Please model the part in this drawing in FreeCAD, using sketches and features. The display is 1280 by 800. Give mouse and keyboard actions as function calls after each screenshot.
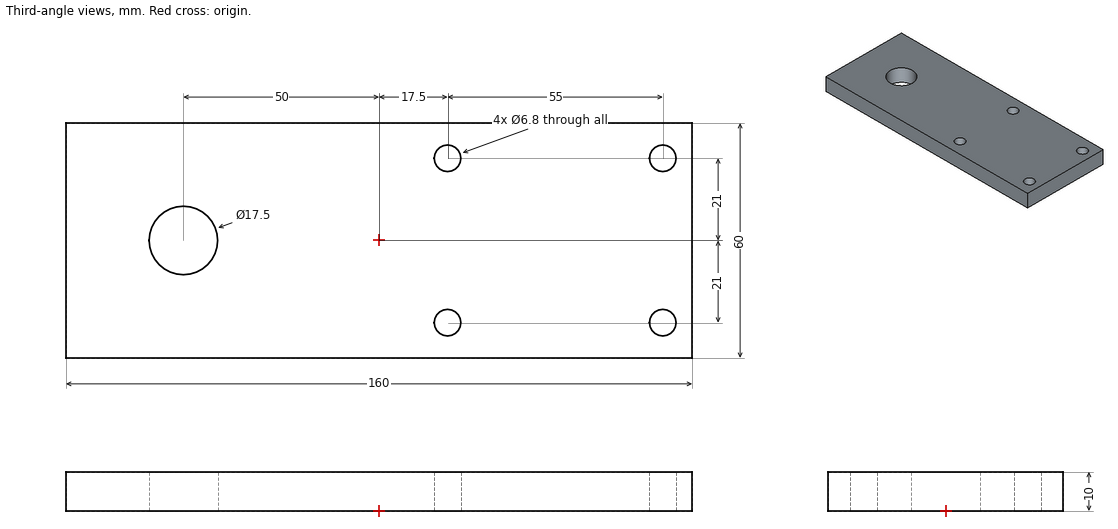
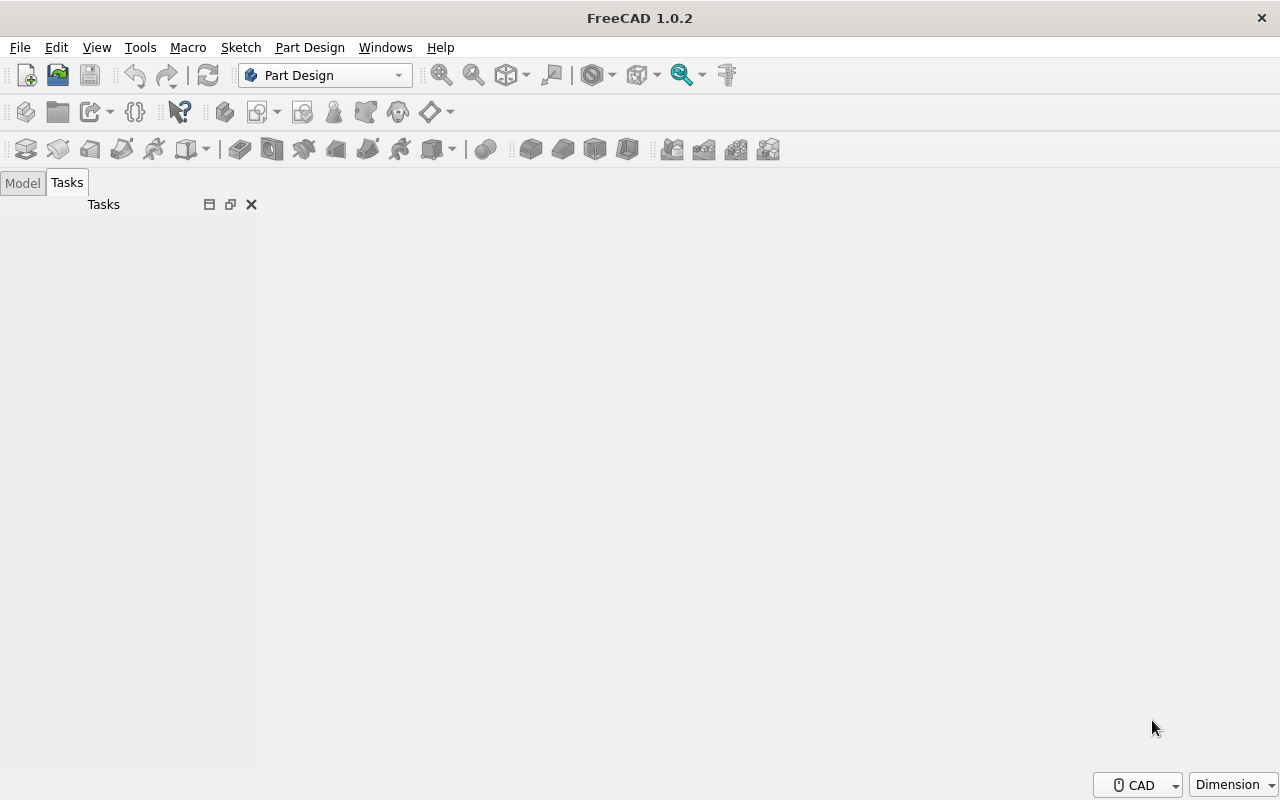
click(26, 76)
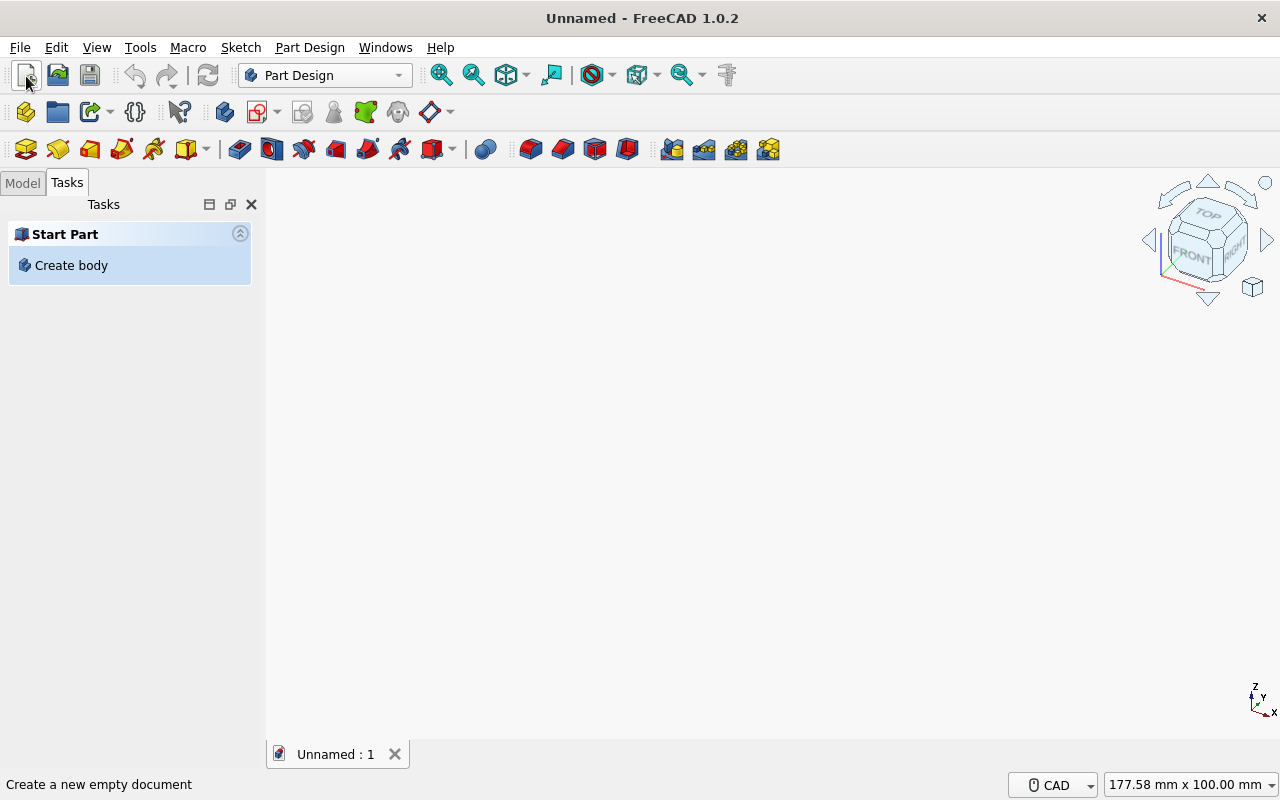
click(258, 112)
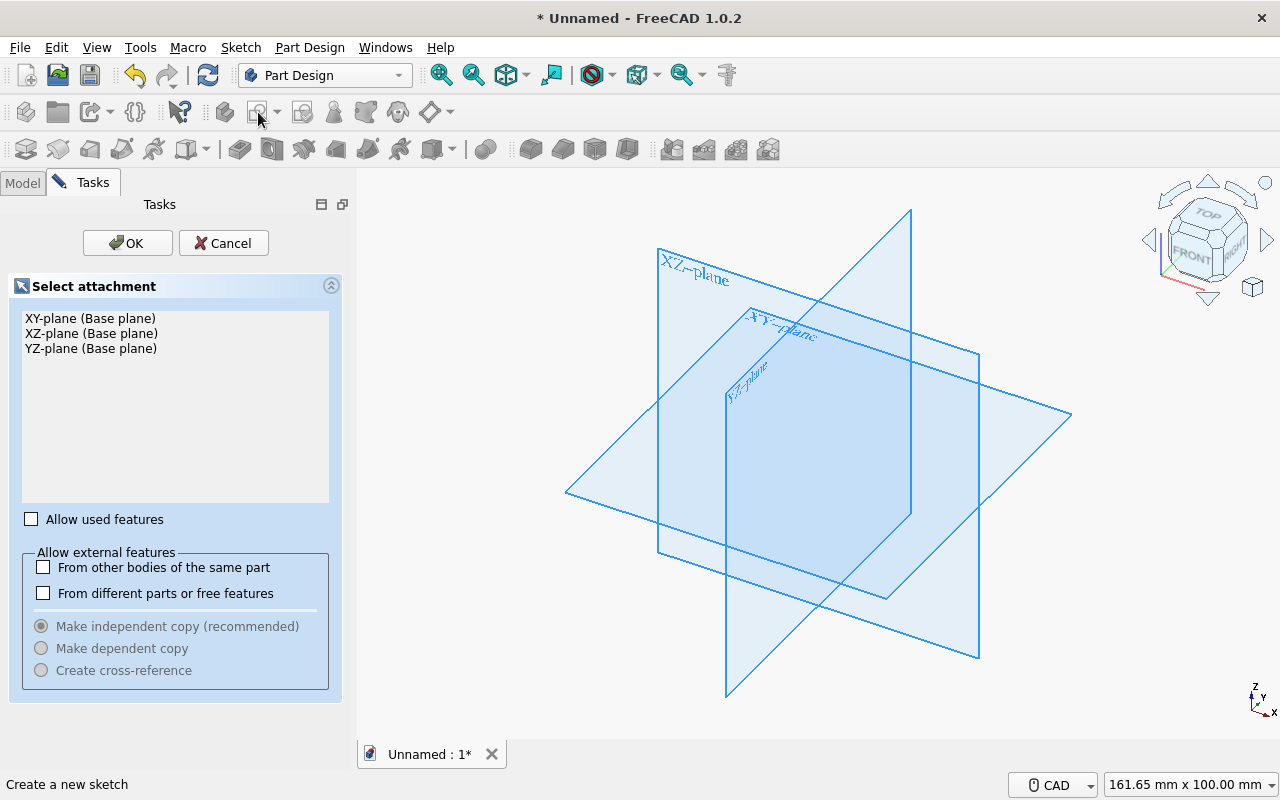
click(82, 318)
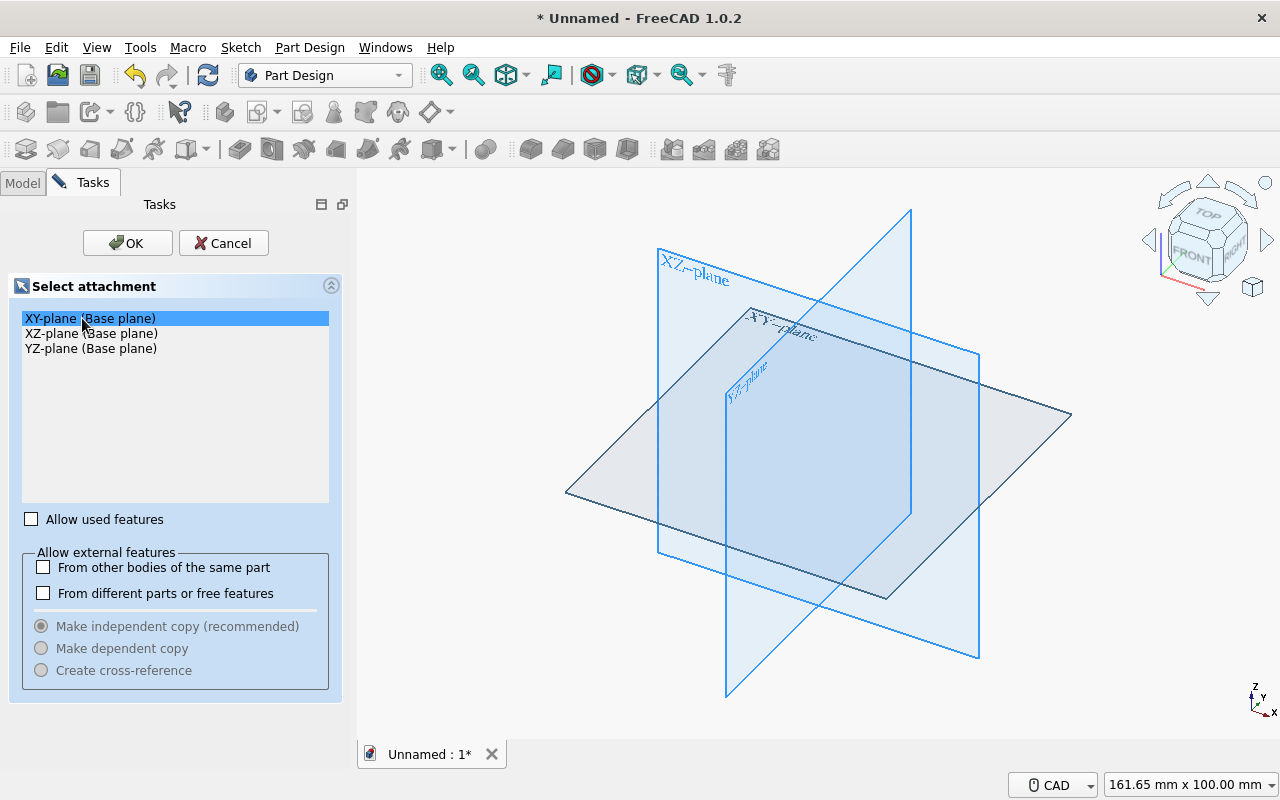
click(128, 243)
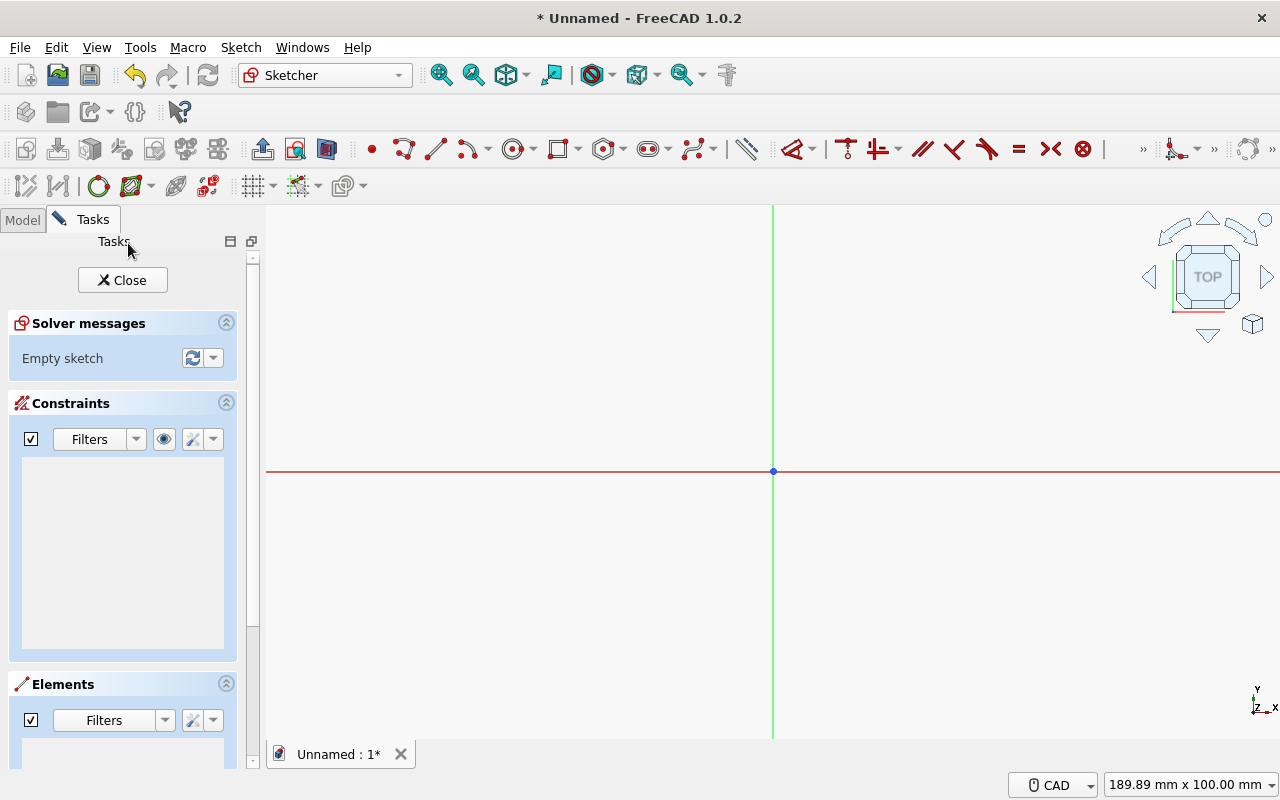
scroll(565, 472, down, 2)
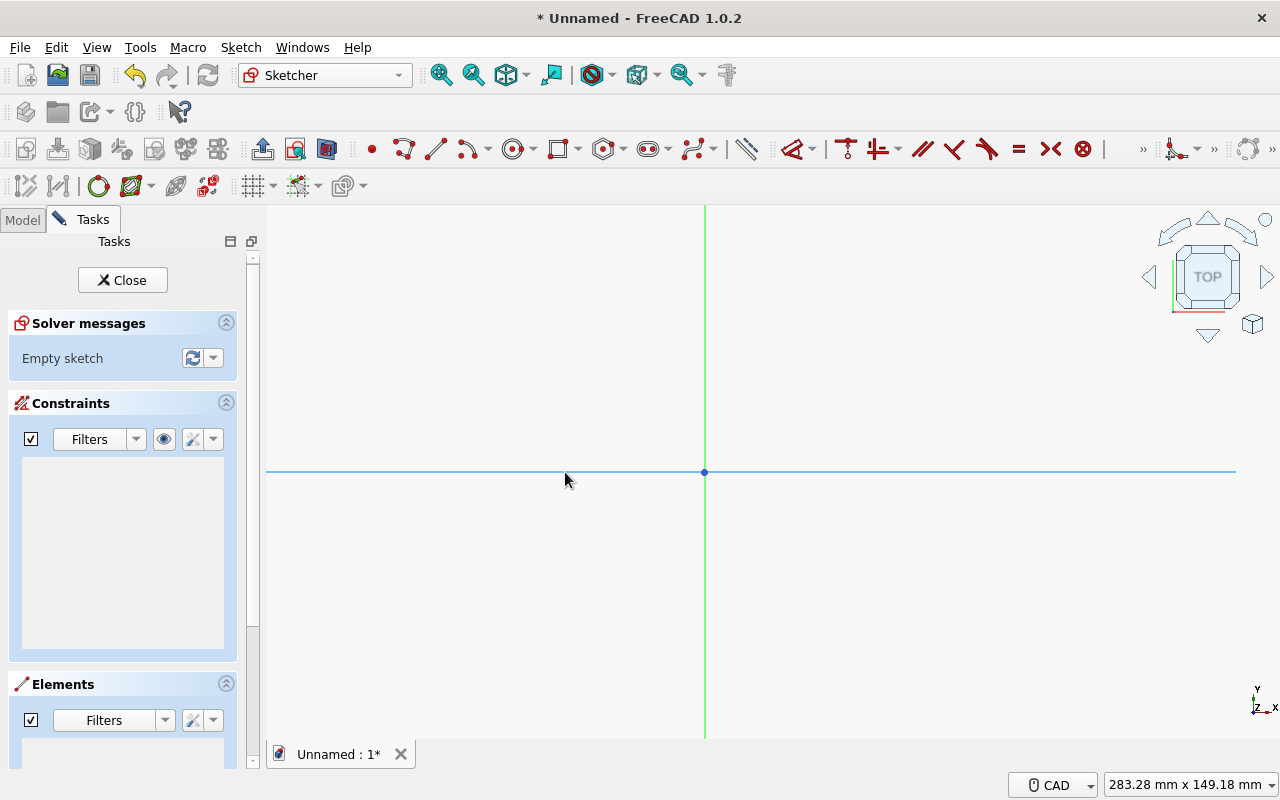
key(g)
key(v)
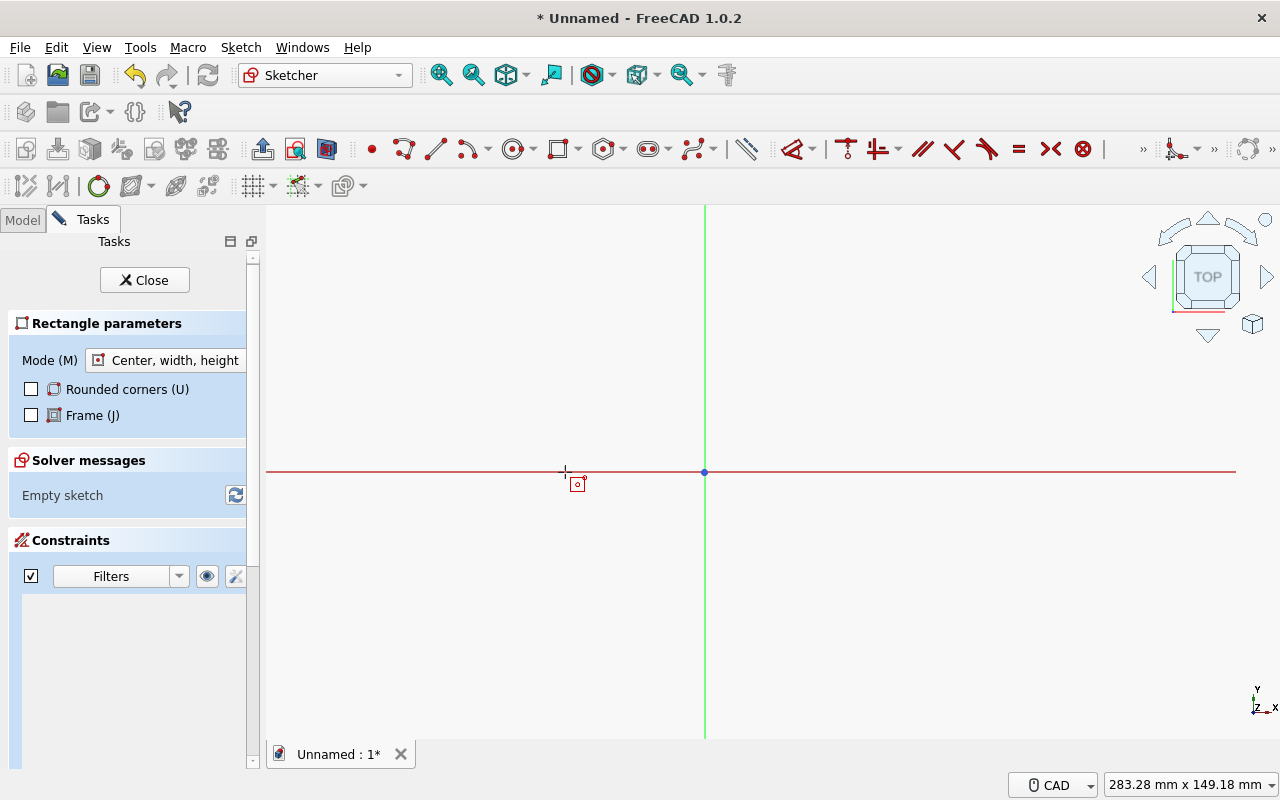
click(705, 472)
click(991, 365)
key(Escape)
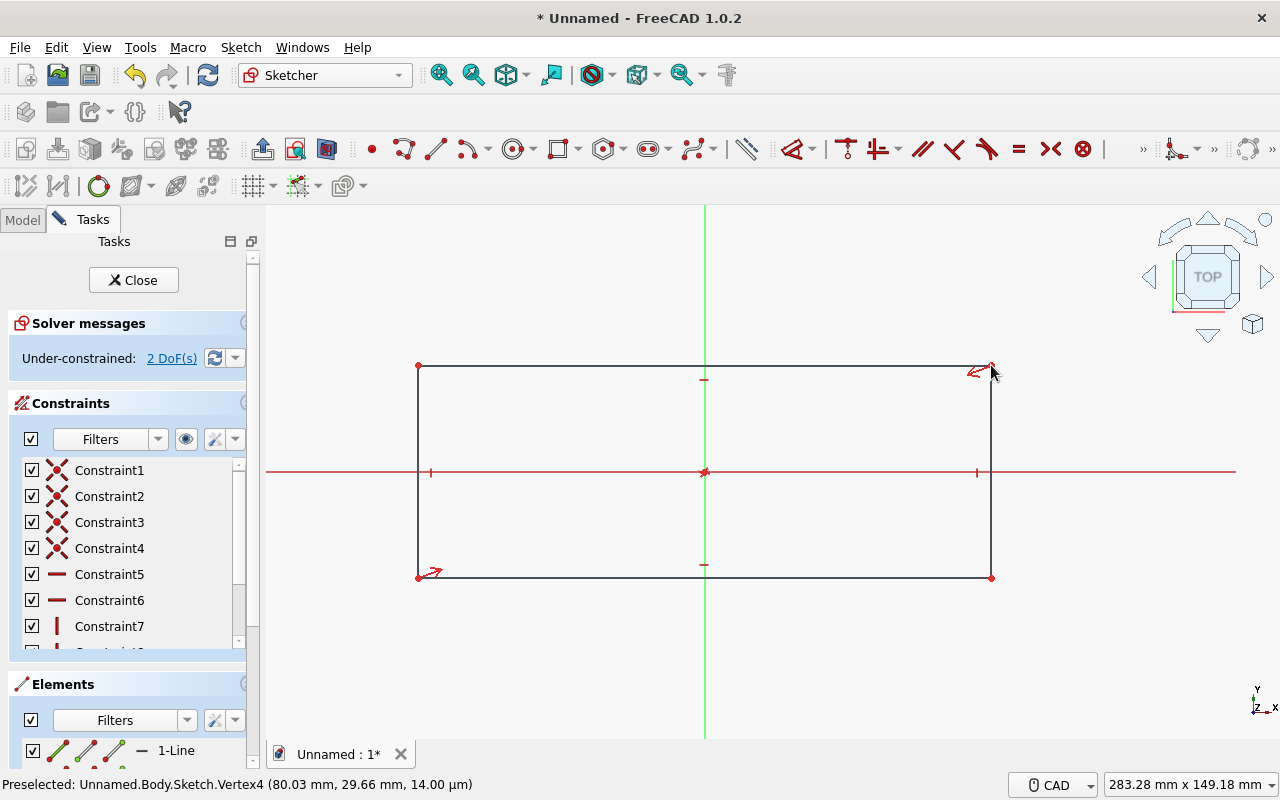
key(d)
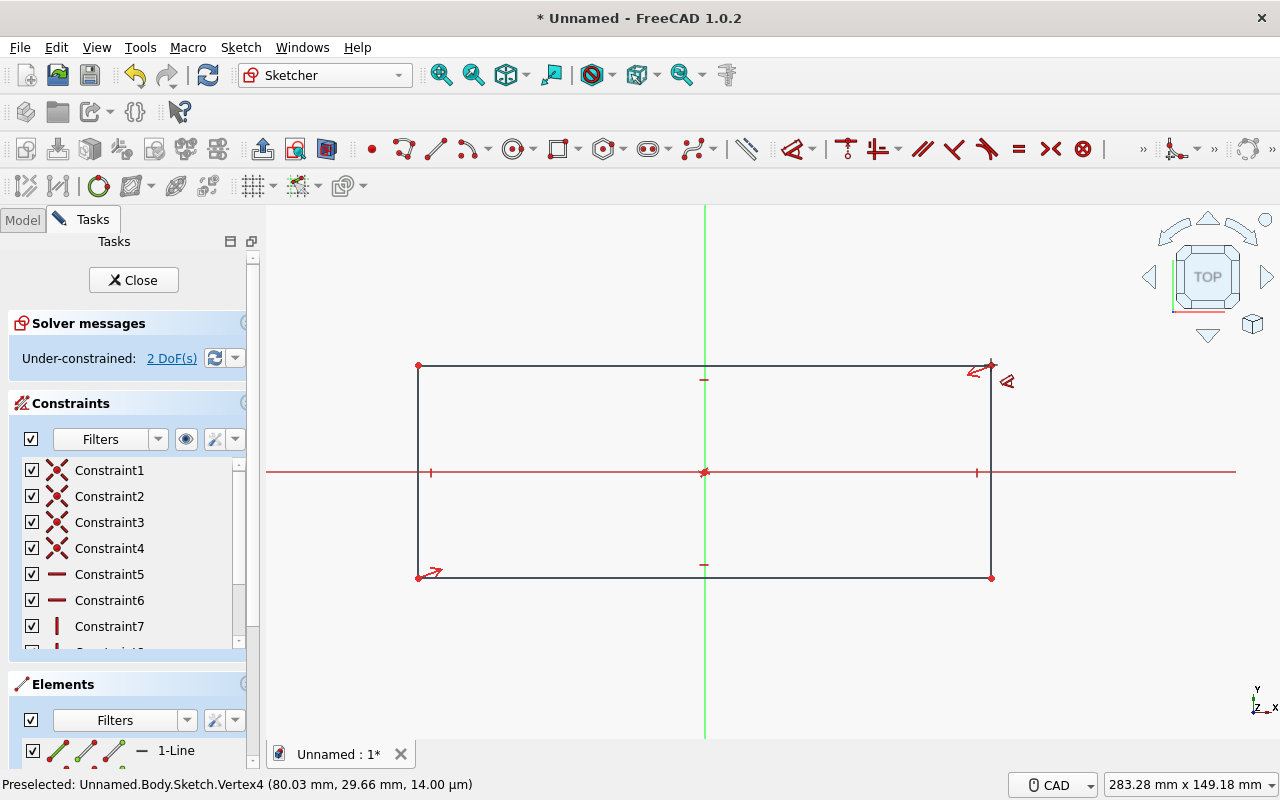
click(991, 515)
click(1025, 423)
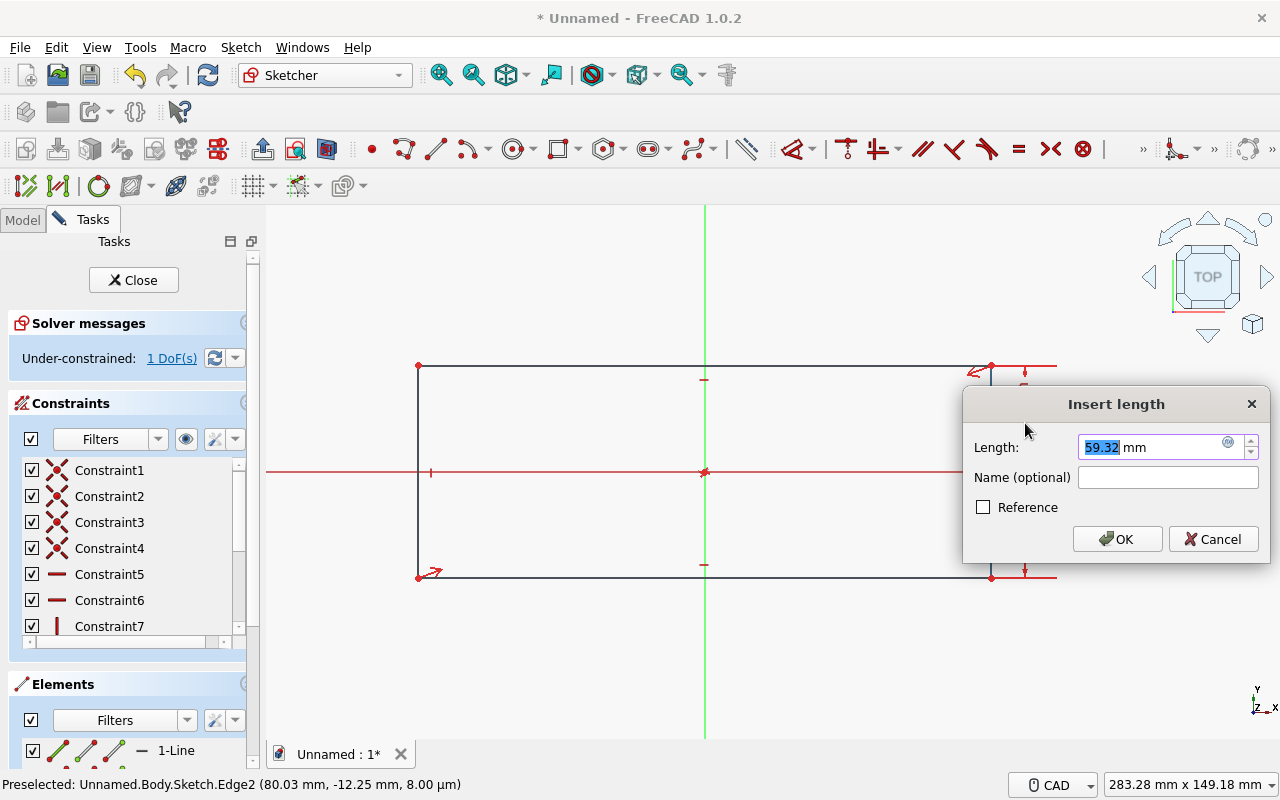
text(60)
key(Return)